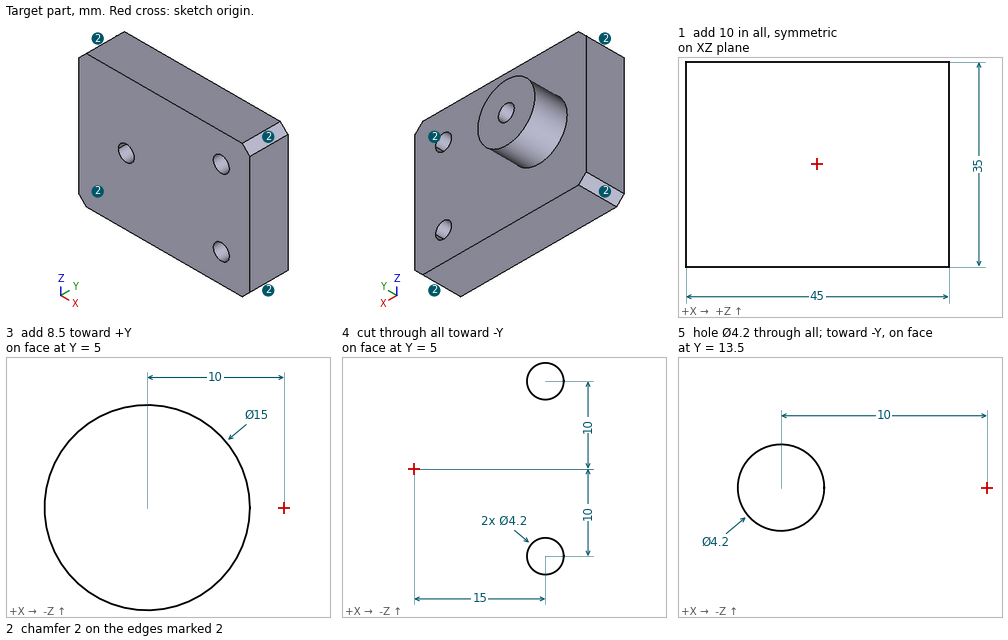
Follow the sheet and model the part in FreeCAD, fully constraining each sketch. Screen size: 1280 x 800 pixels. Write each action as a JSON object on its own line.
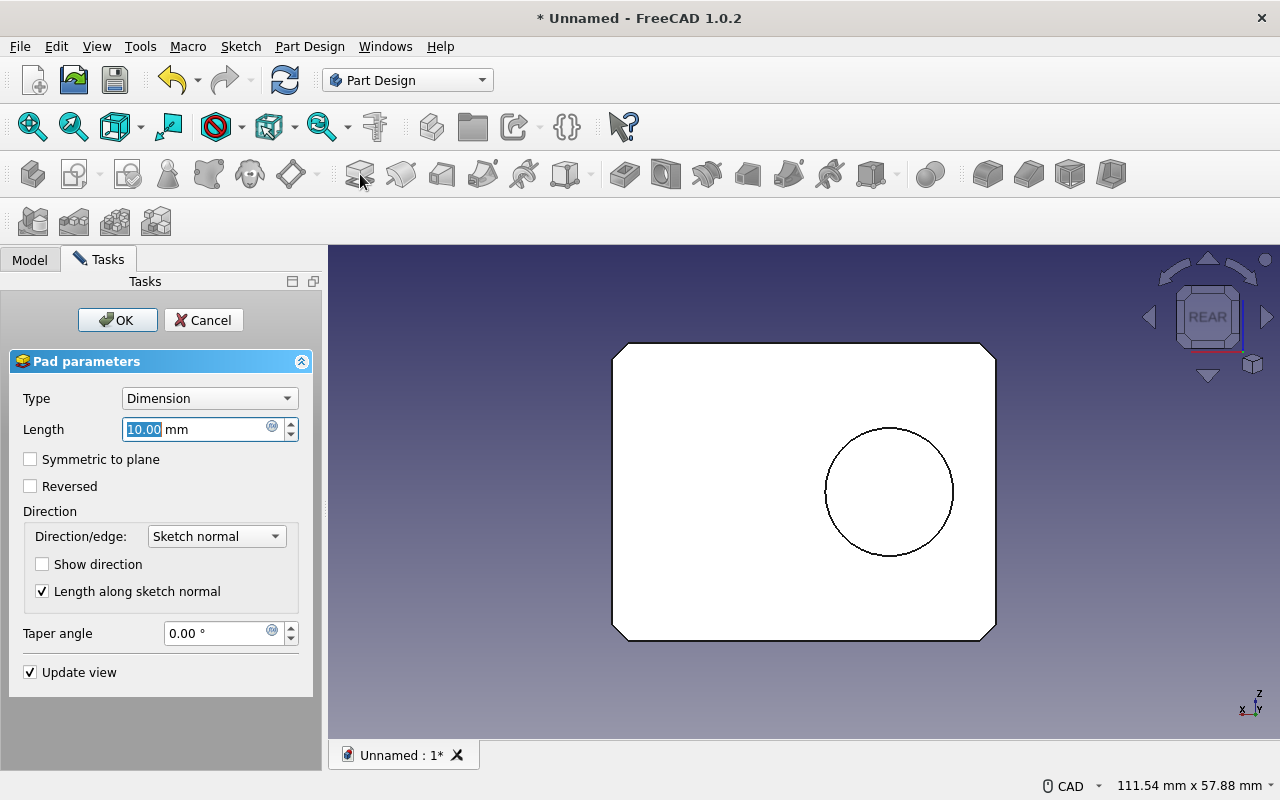
{"action": "type", "text": "8.5"}
{"action": "key", "text": "Tab"}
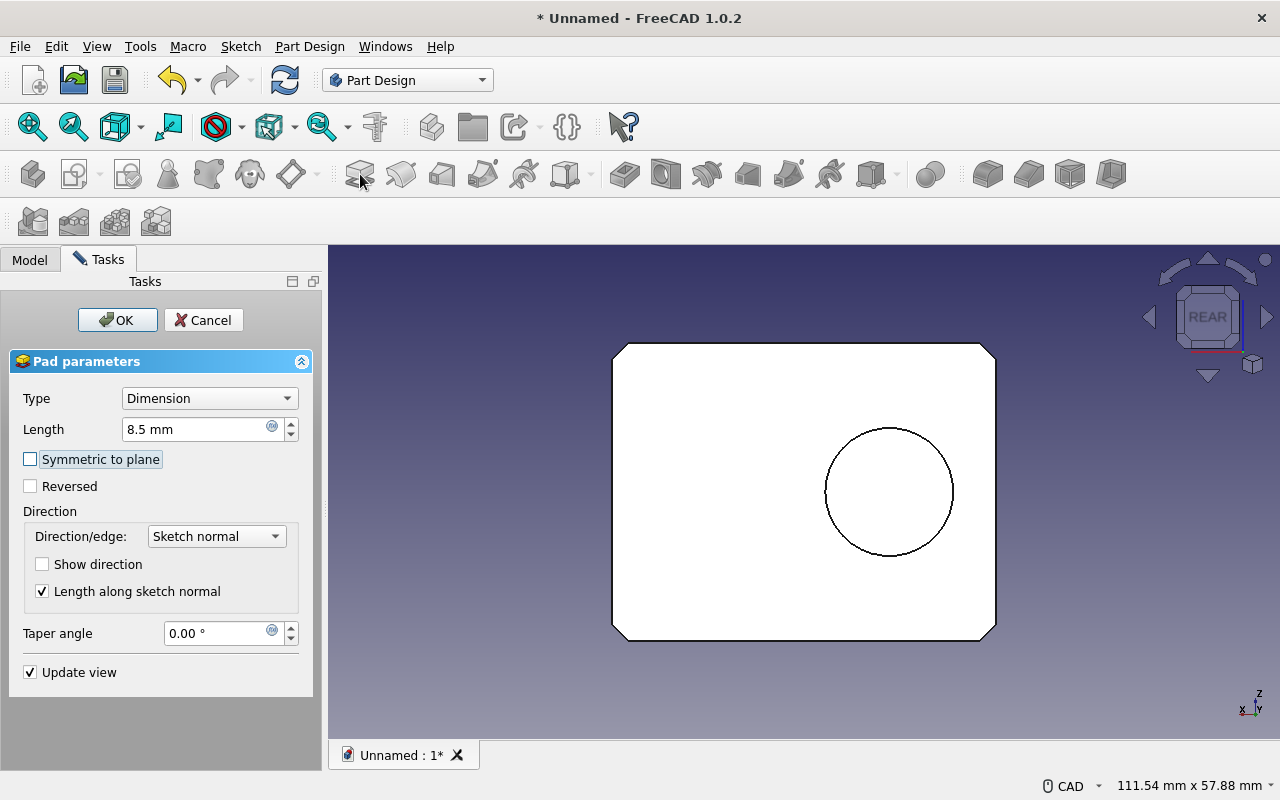
{"action": "left_click", "coordinate": [118, 320]}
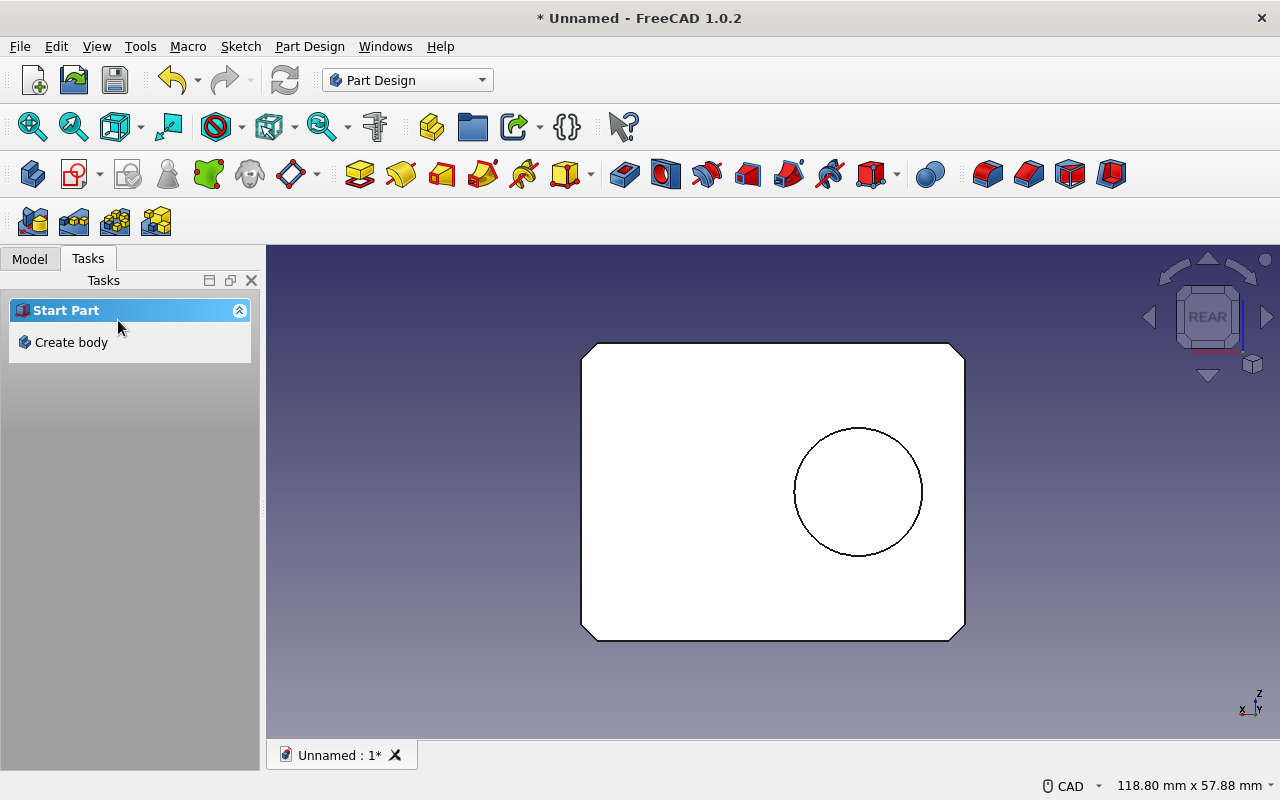
{"action": "left_click", "coordinate": [718, 534]}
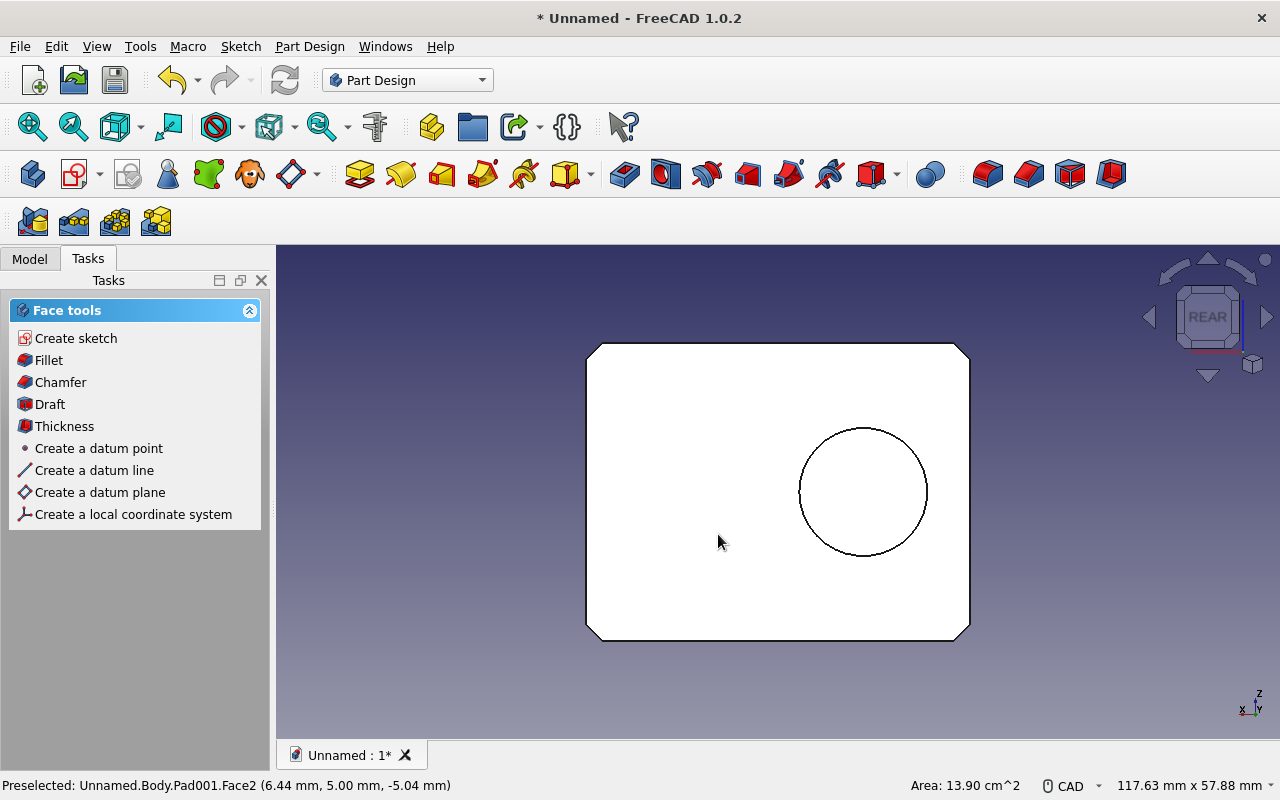
{"action": "left_click", "coordinate": [74, 174]}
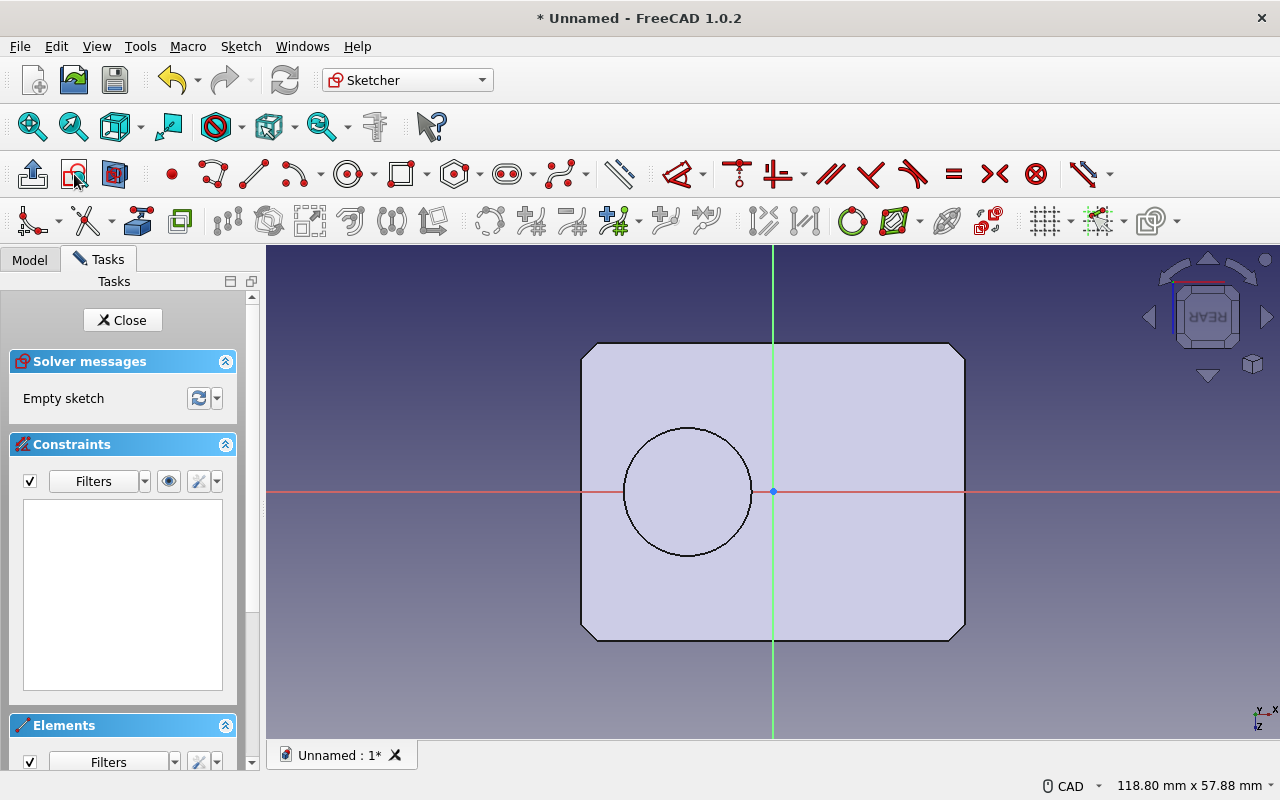
{"action": "left_click", "coordinate": [115, 174]}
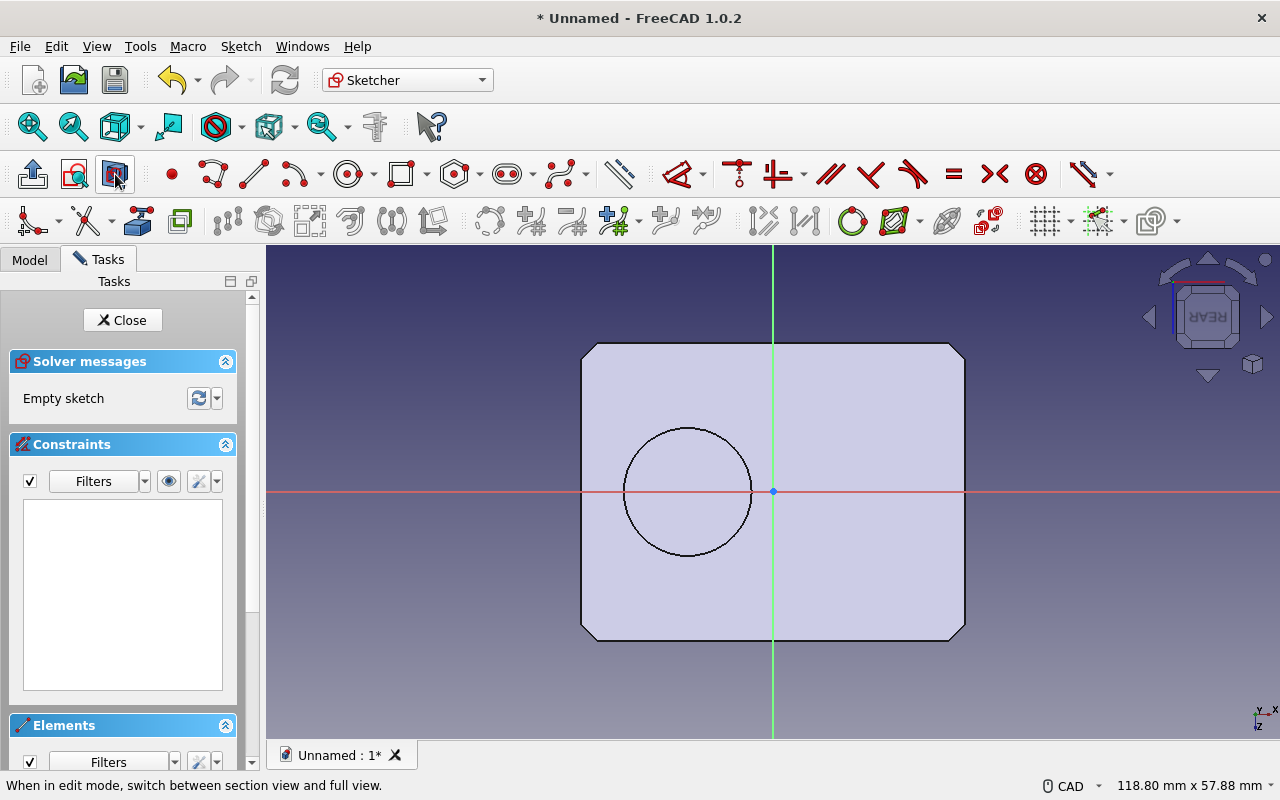
{"action": "scroll", "coordinate": [1115, 492], "scroll_direction": "up", "scroll_amount": 2}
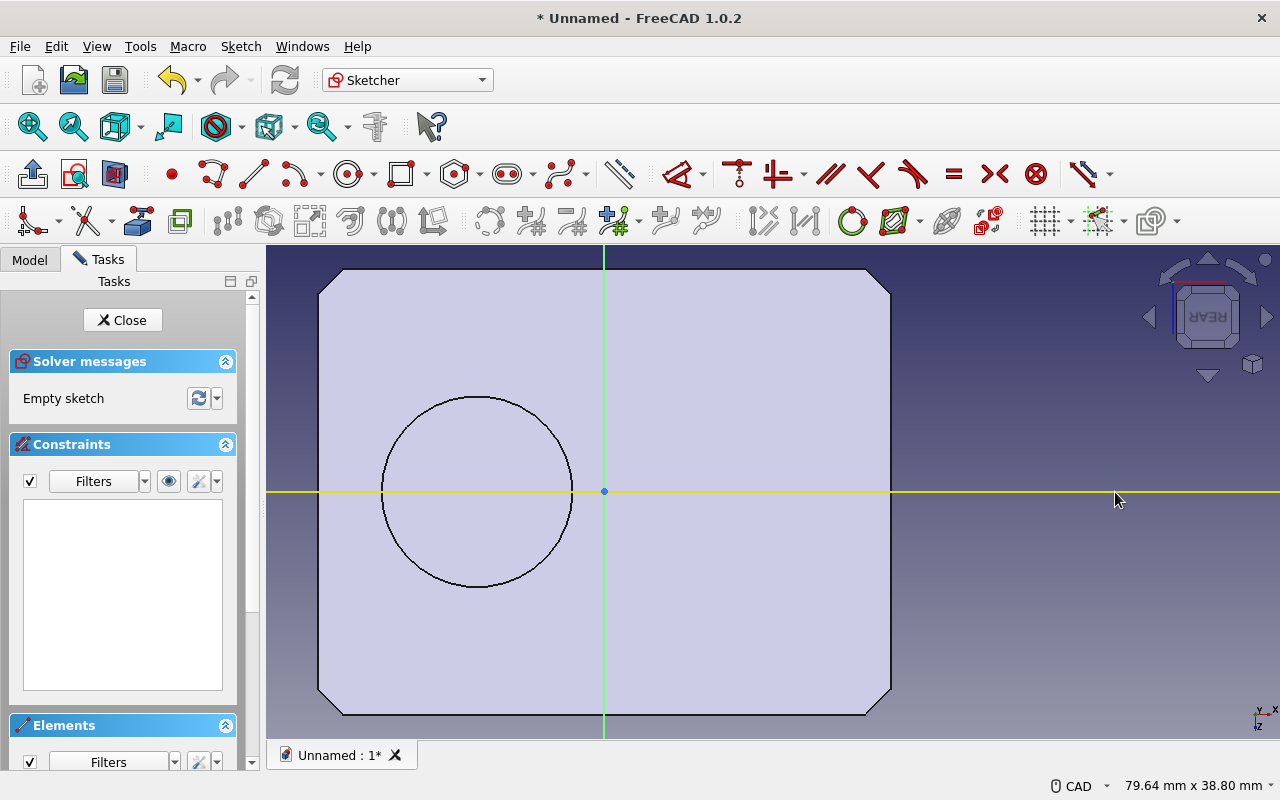
{"action": "key", "text": "g c"}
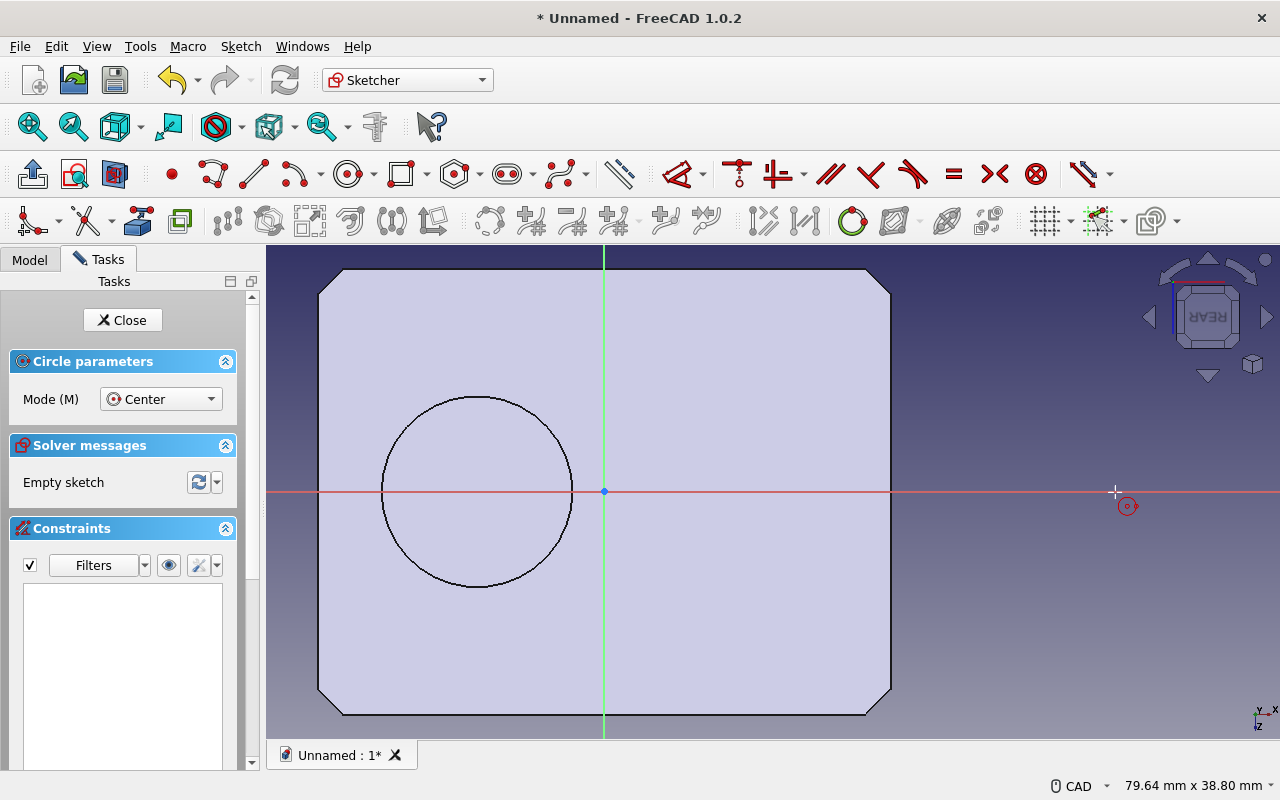
{"action": "left_click", "coordinate": [795, 619]}
{"action": "mouse_move", "coordinate": [814, 600]}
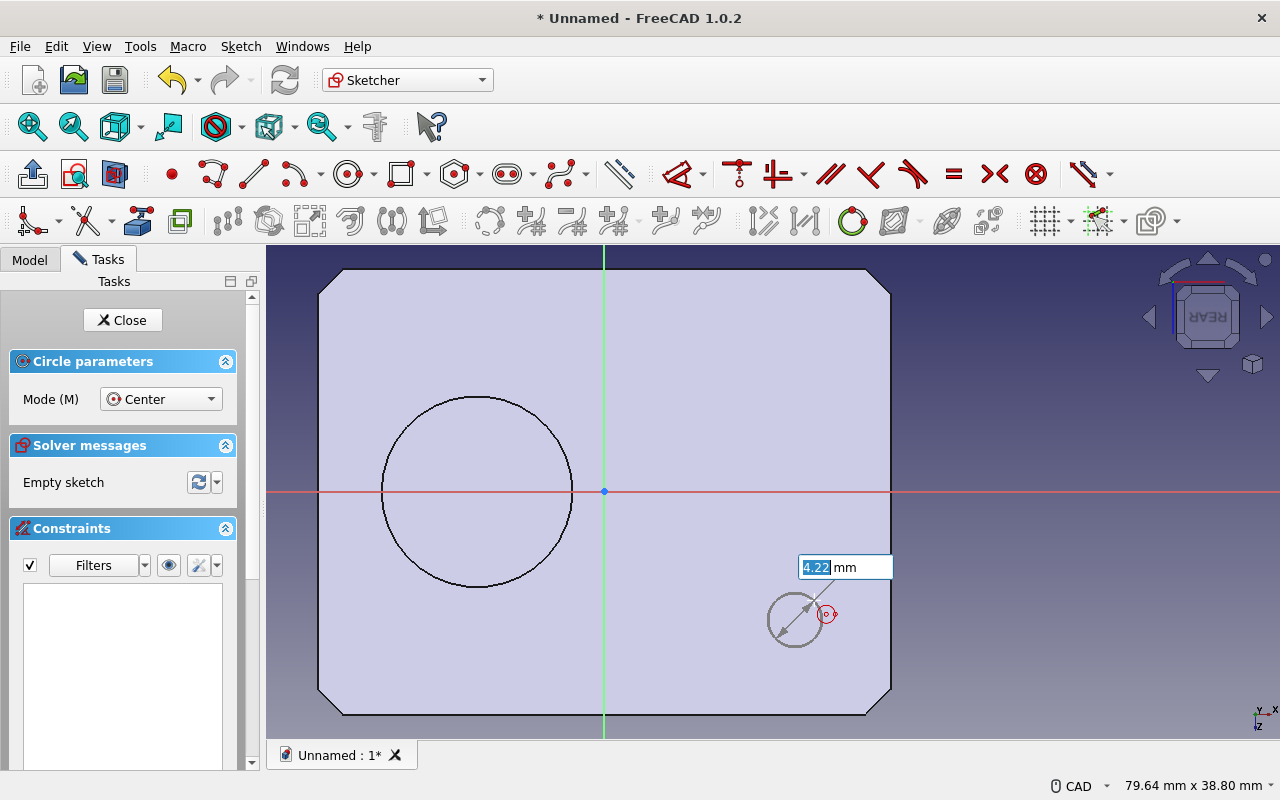
{"action": "type", "text": "4.2"}
{"action": "key", "text": "Return"}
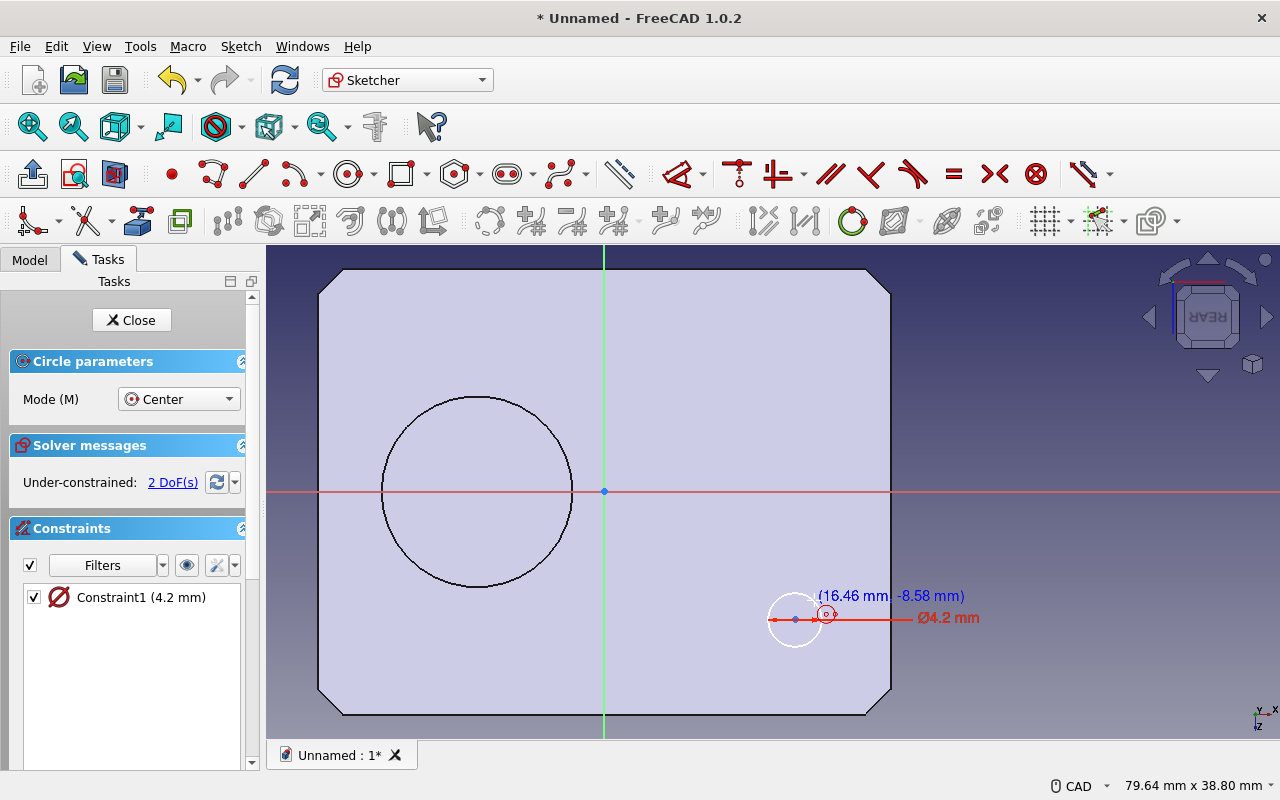
{"action": "left_click", "coordinate": [795, 364]}
{"action": "mouse_move", "coordinate": [814, 346]}